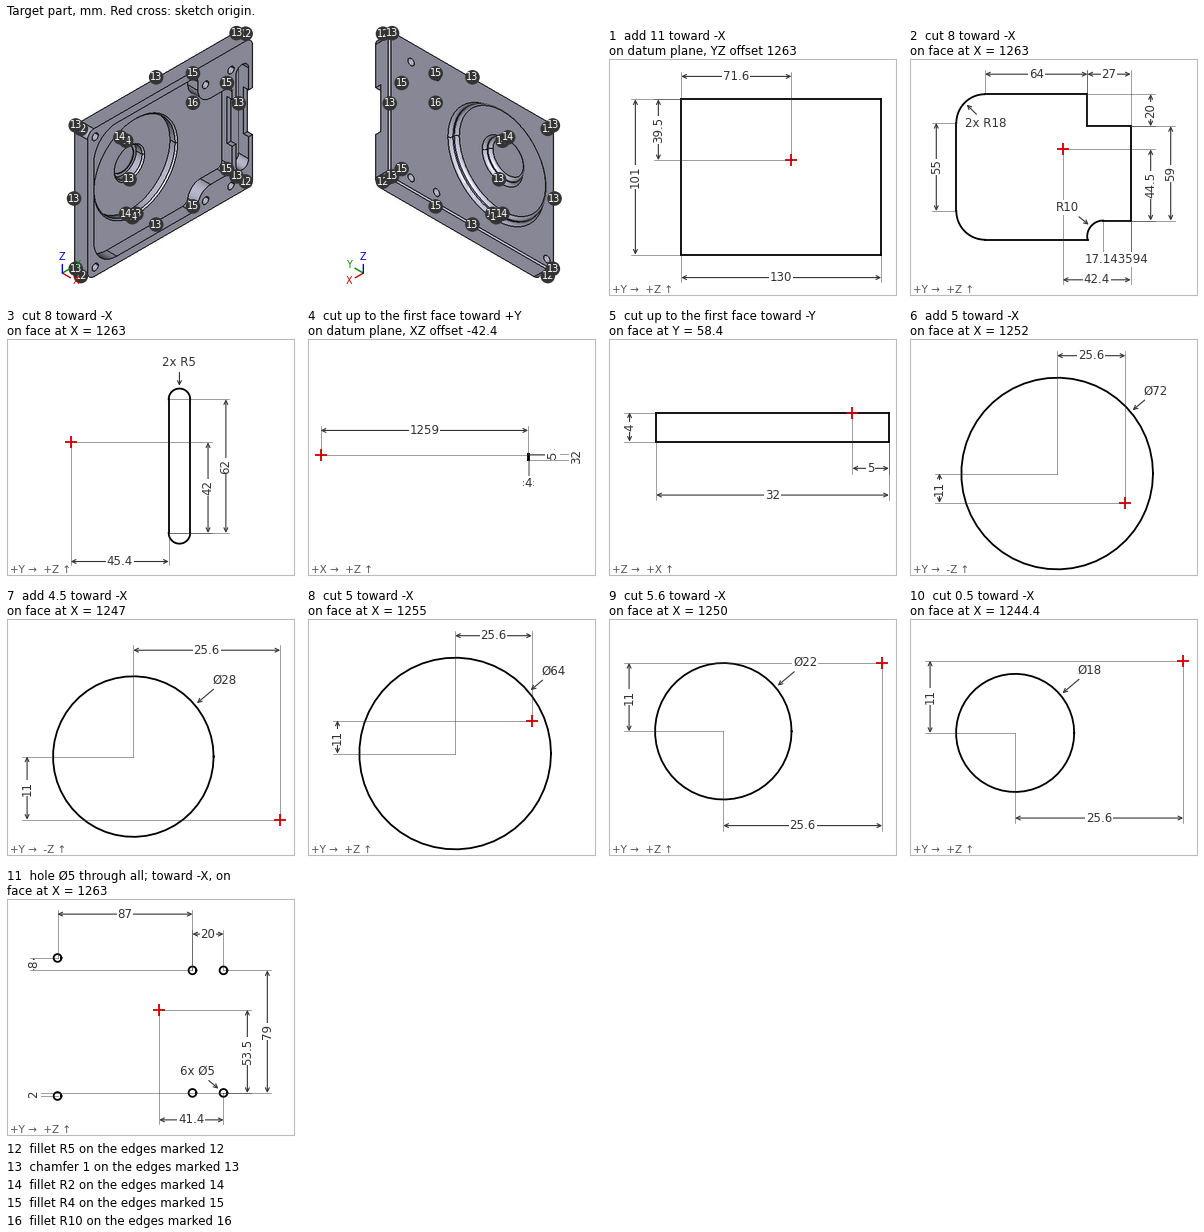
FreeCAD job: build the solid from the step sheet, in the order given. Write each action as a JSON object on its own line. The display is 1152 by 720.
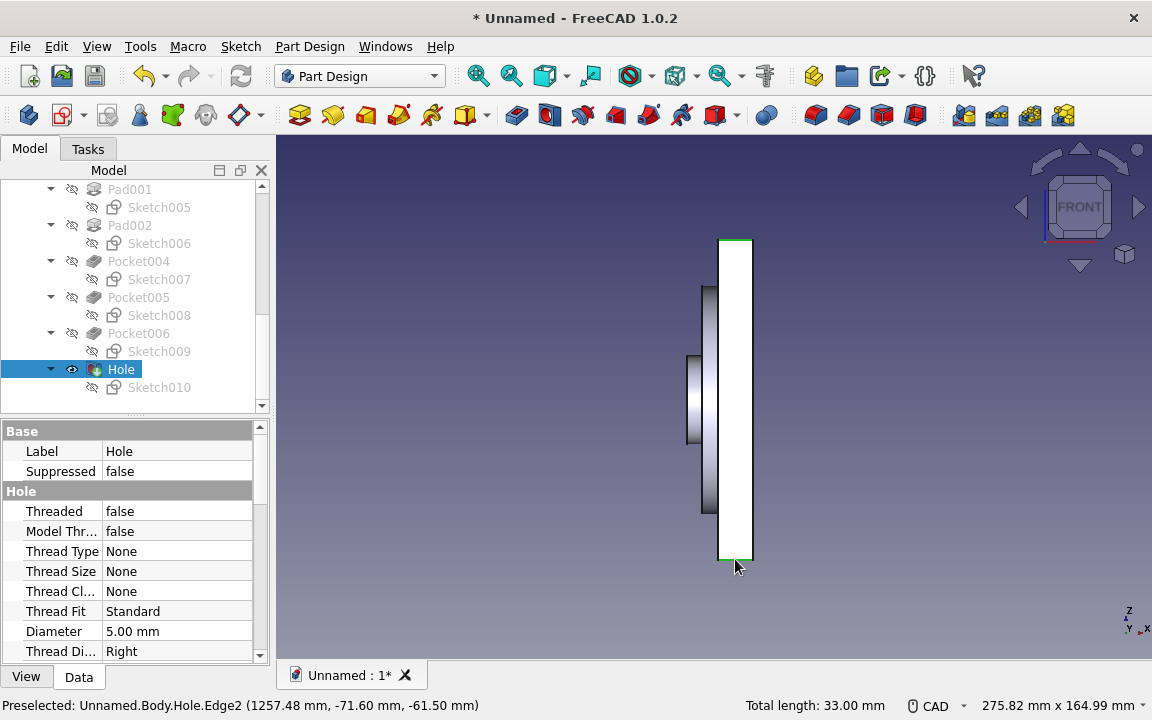
{"action": "key", "text": "3"}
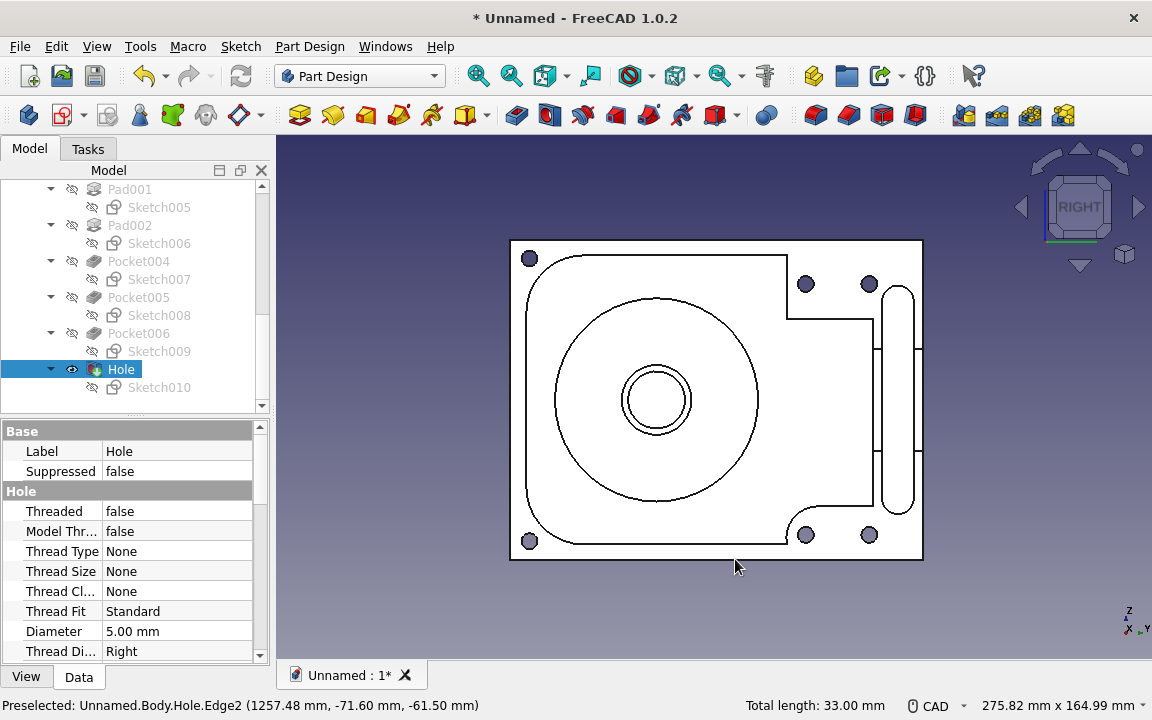
{"action": "key", "text": "5"}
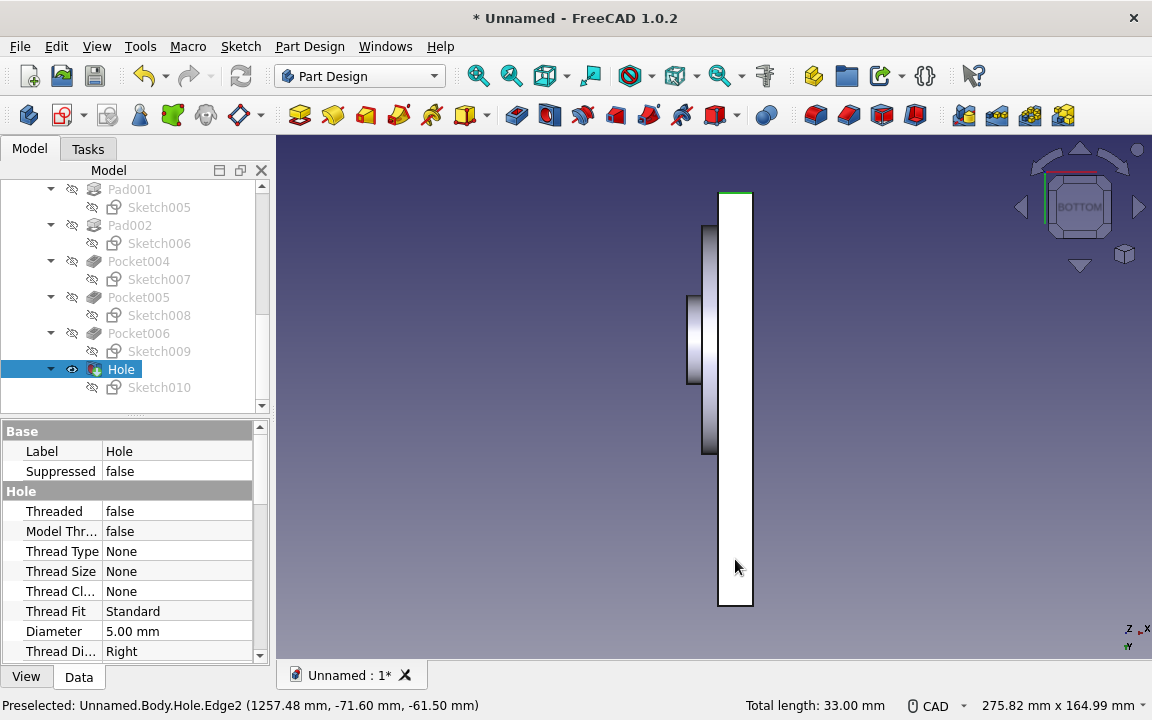
{"action": "left_click", "coordinate": [735, 605], "text": "ctrl"}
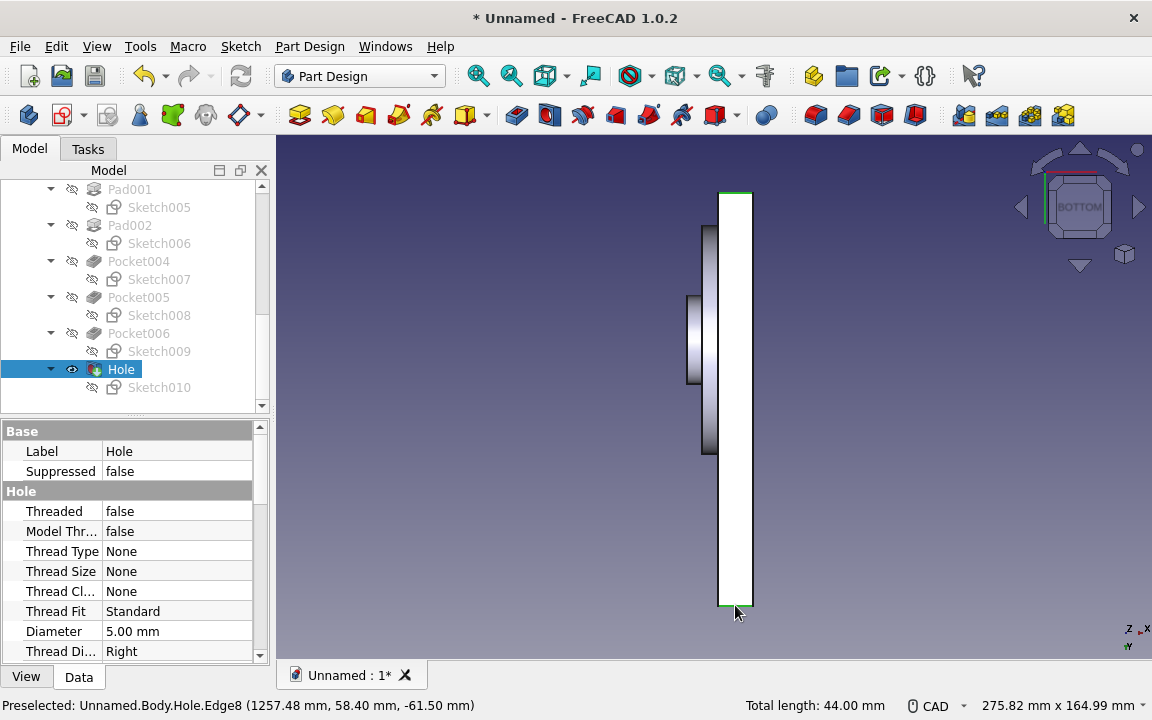
{"action": "left_click", "coordinate": [816, 116]}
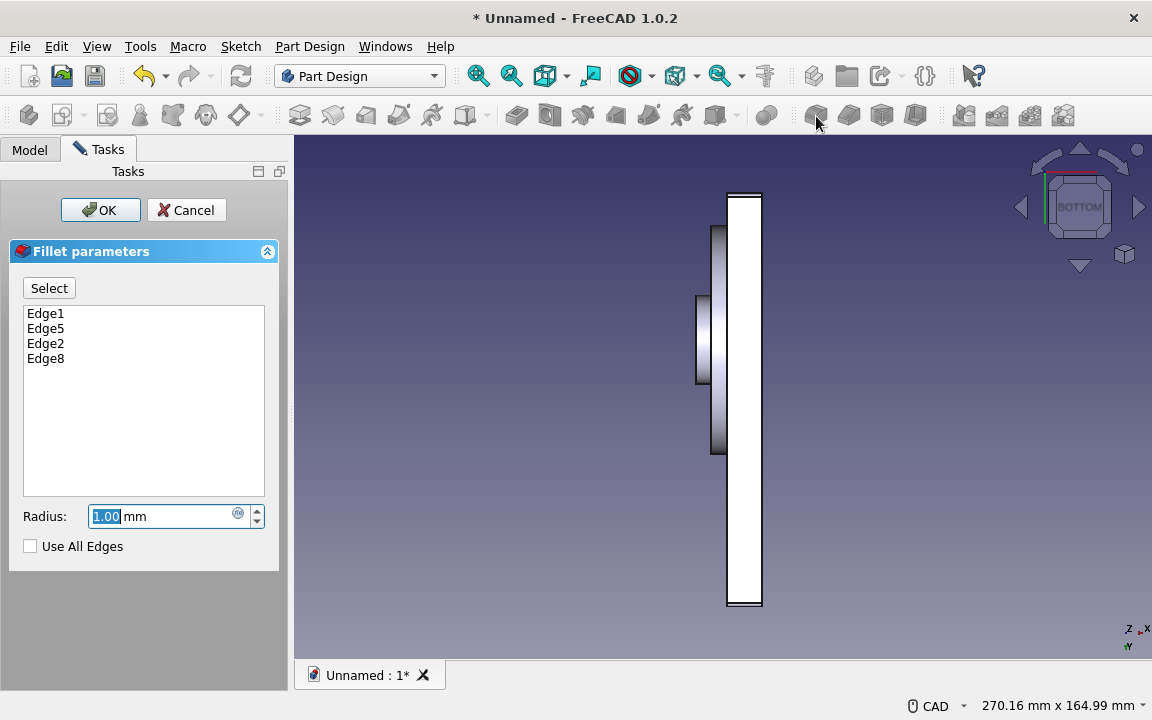
{"action": "type", "text": "5"}
{"action": "key", "text": "Tab"}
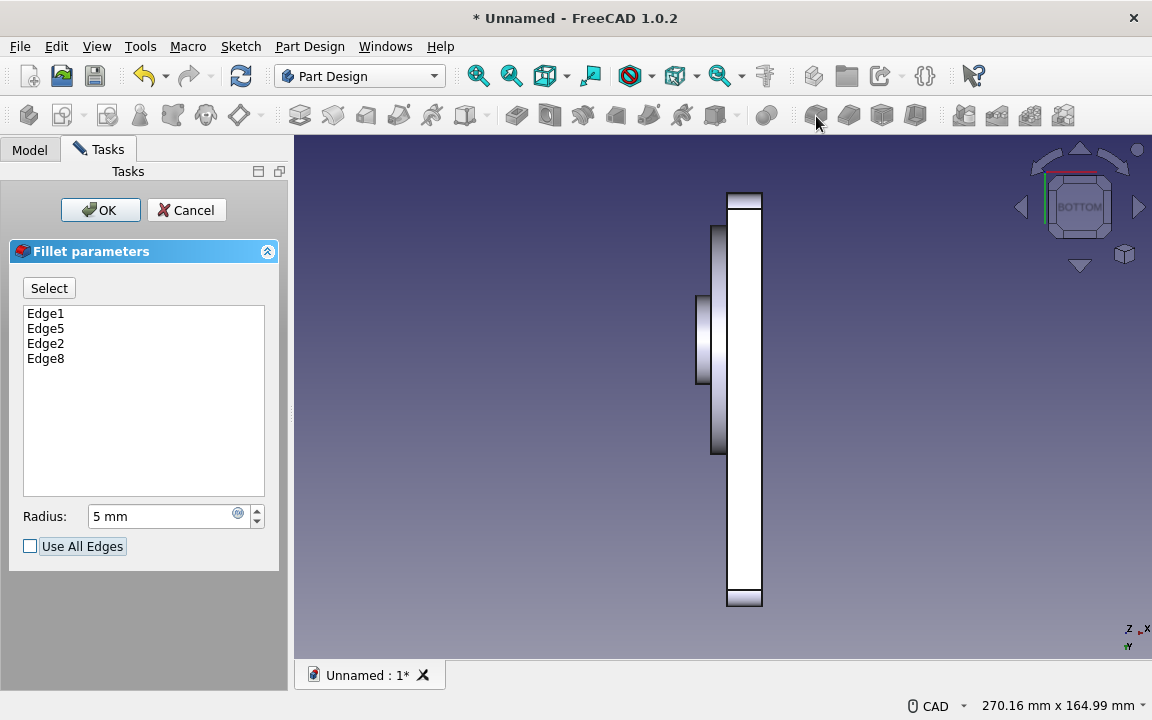
{"action": "left_click", "coordinate": [101, 210]}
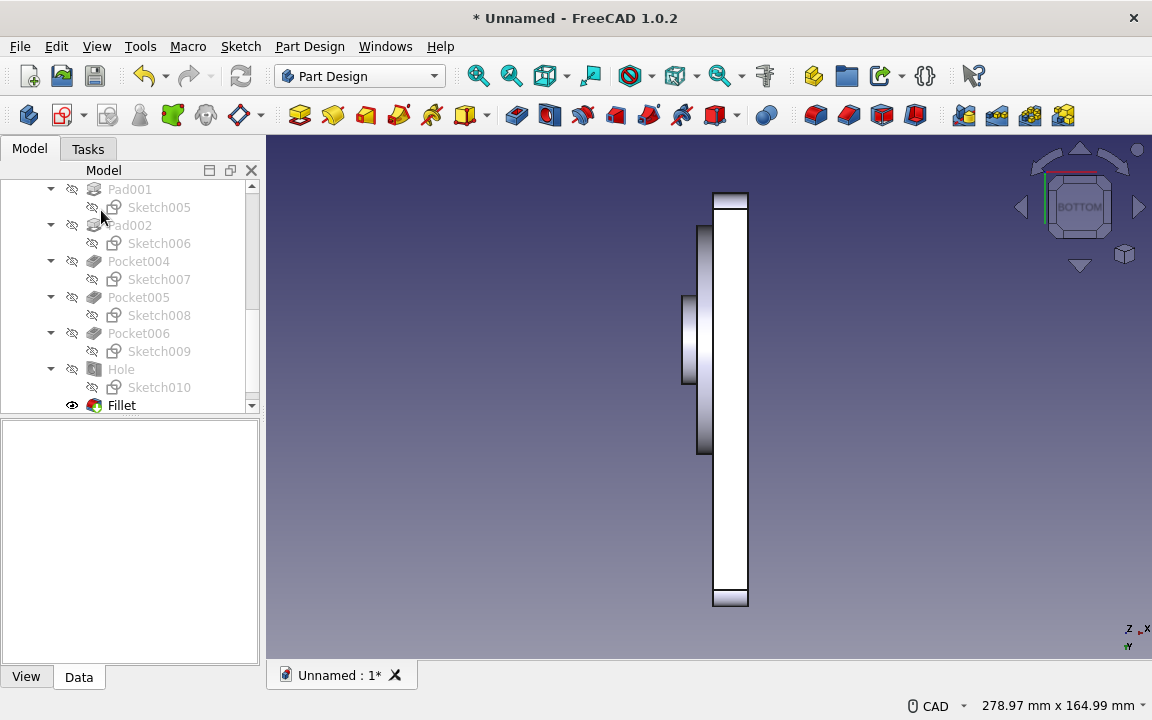
{"action": "left_click", "coordinate": [713, 399]}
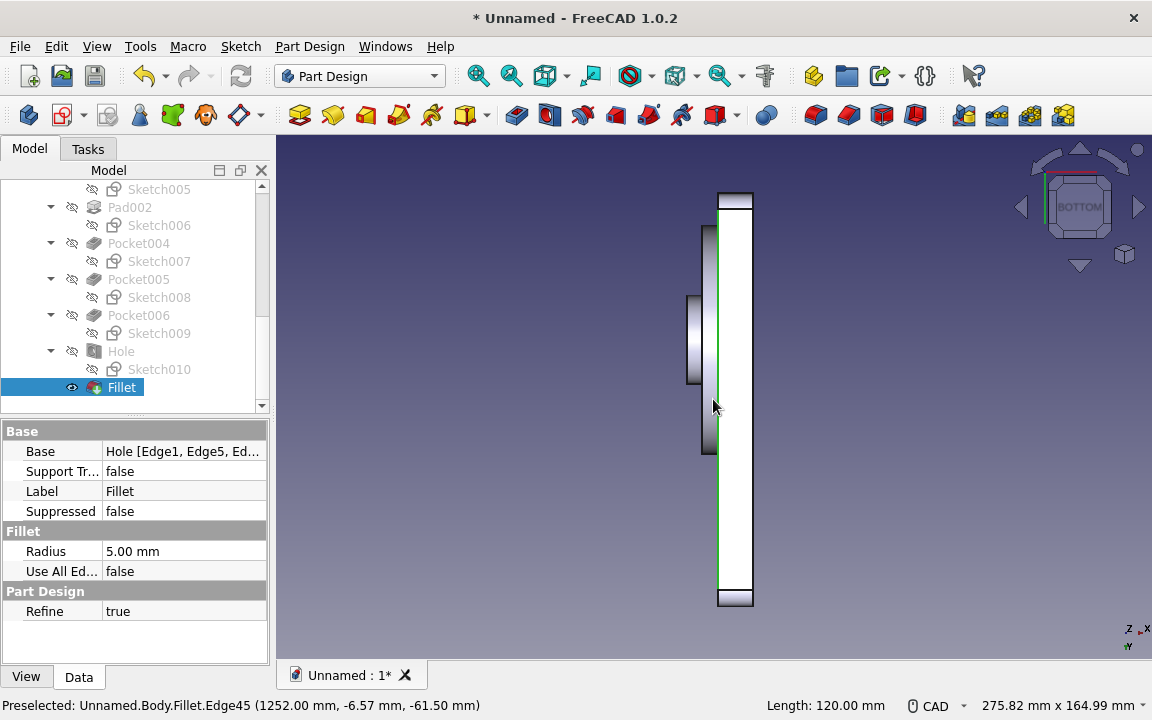
{"action": "left_click", "coordinate": [718, 197], "text": "ctrl"}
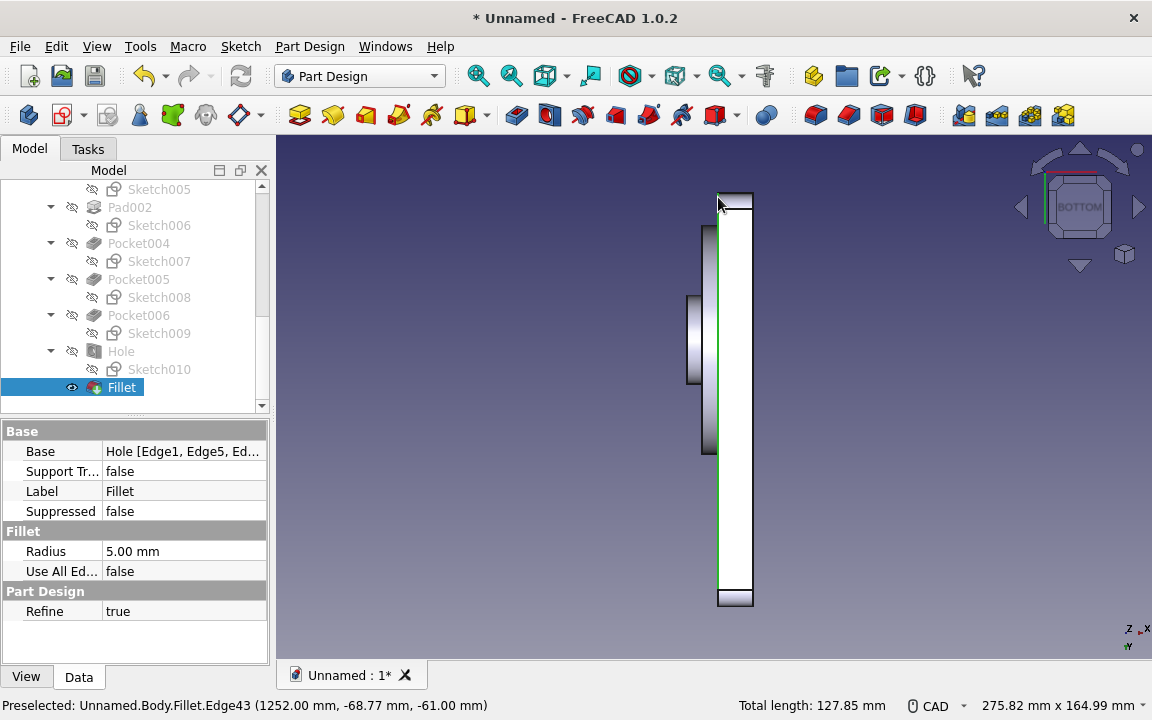
{"action": "left_click", "coordinate": [718, 601], "text": "ctrl"}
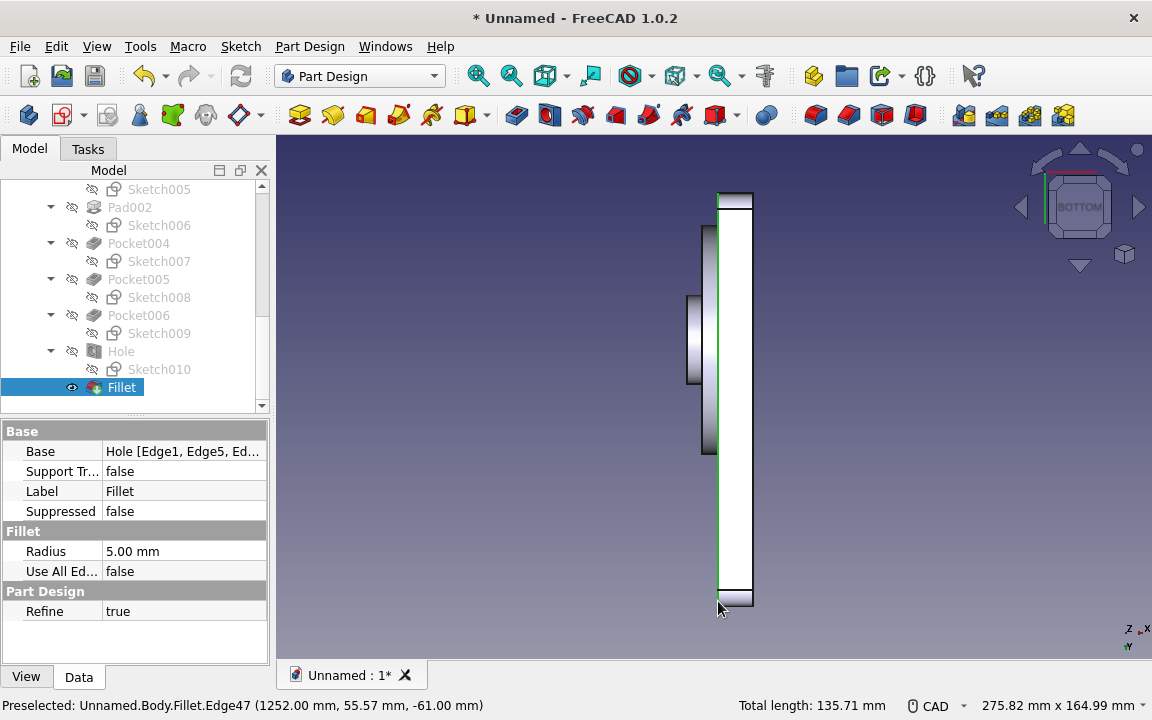
{"action": "key", "text": "0"}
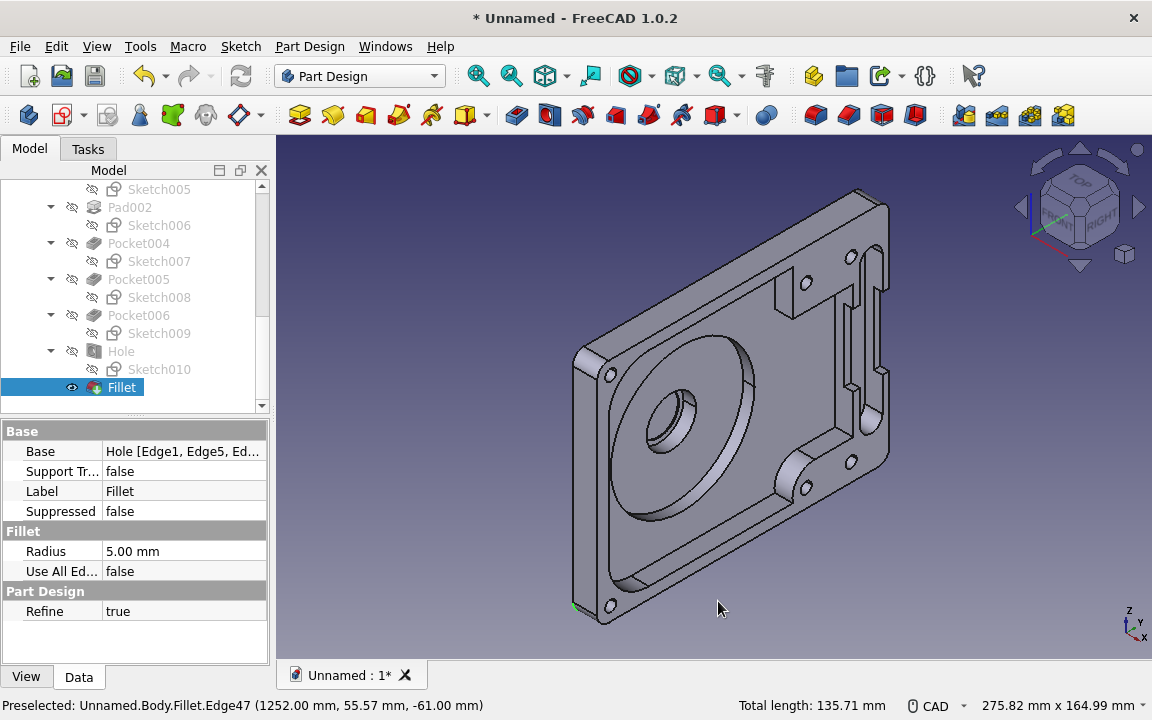
{"action": "left_click", "coordinate": [573, 361], "text": "ctrl"}